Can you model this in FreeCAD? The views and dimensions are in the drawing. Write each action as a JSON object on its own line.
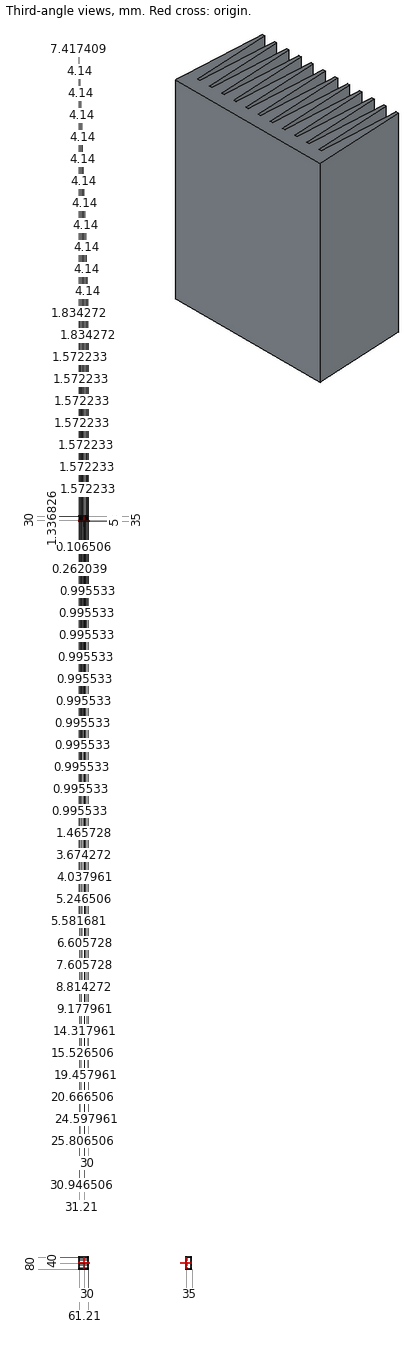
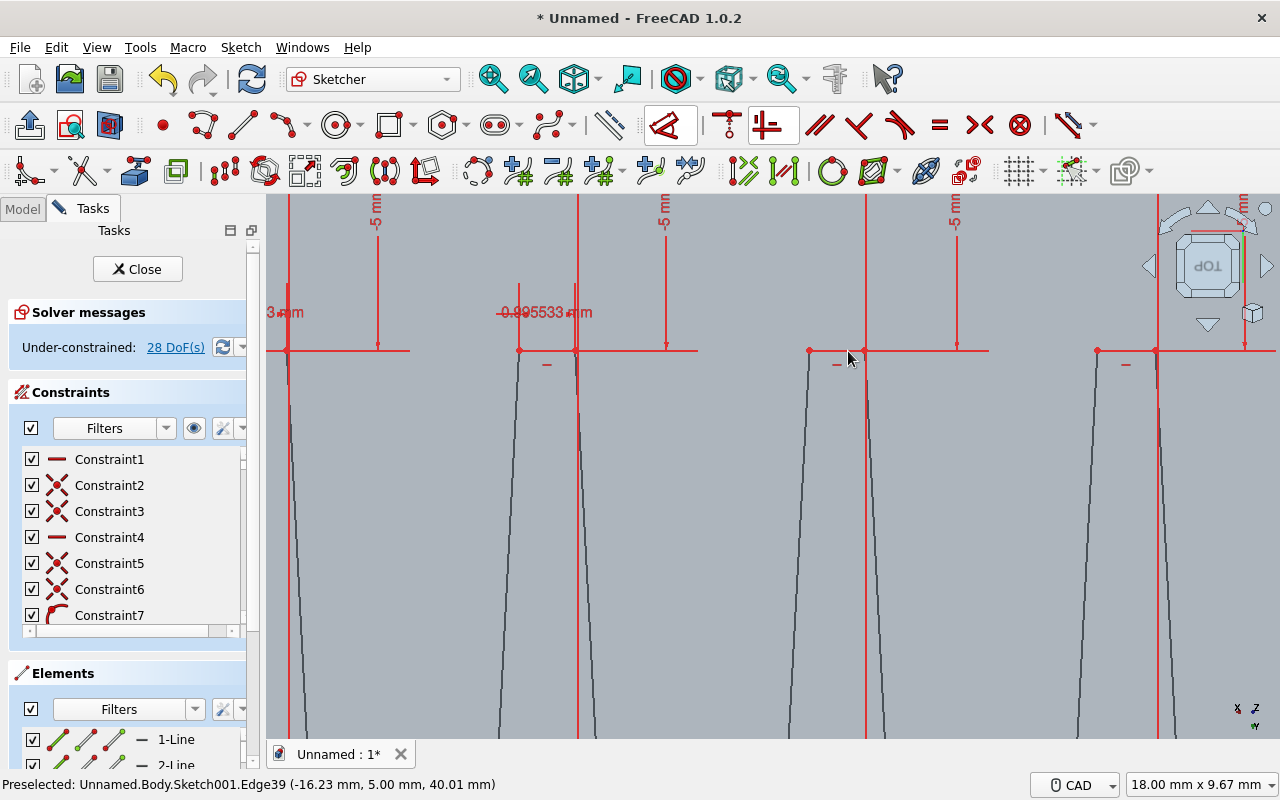
{"action": "key", "text": "l"}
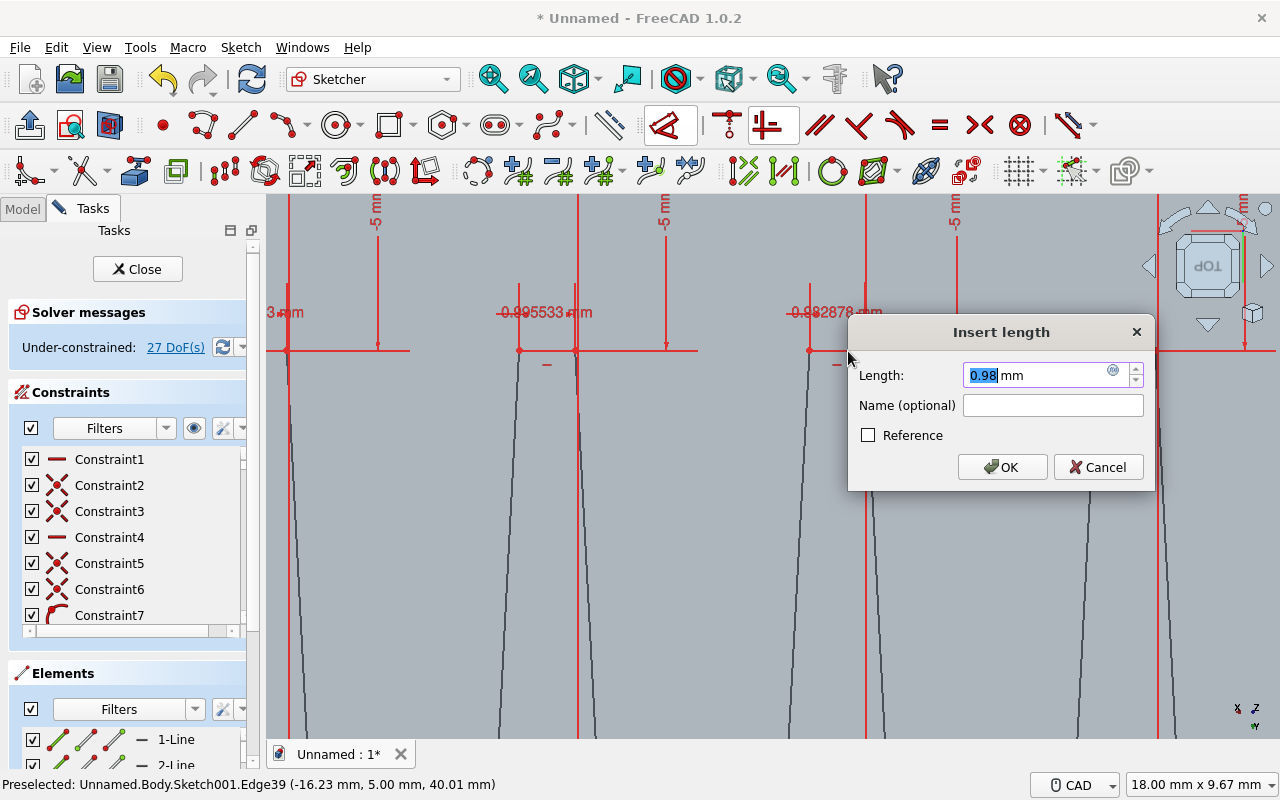
{"action": "type", "text": "0.995533"}
{"action": "key", "text": "Return"}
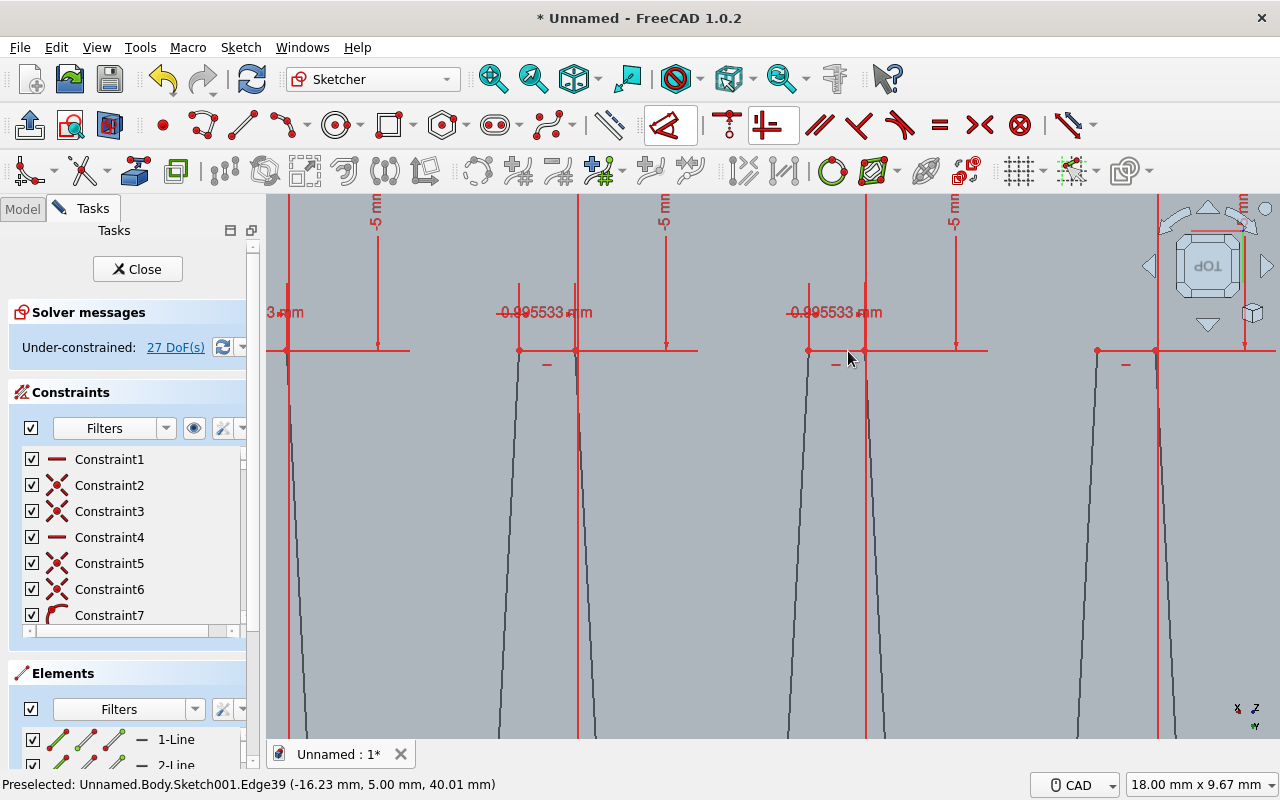
{"action": "left_click", "coordinate": [1115, 351]}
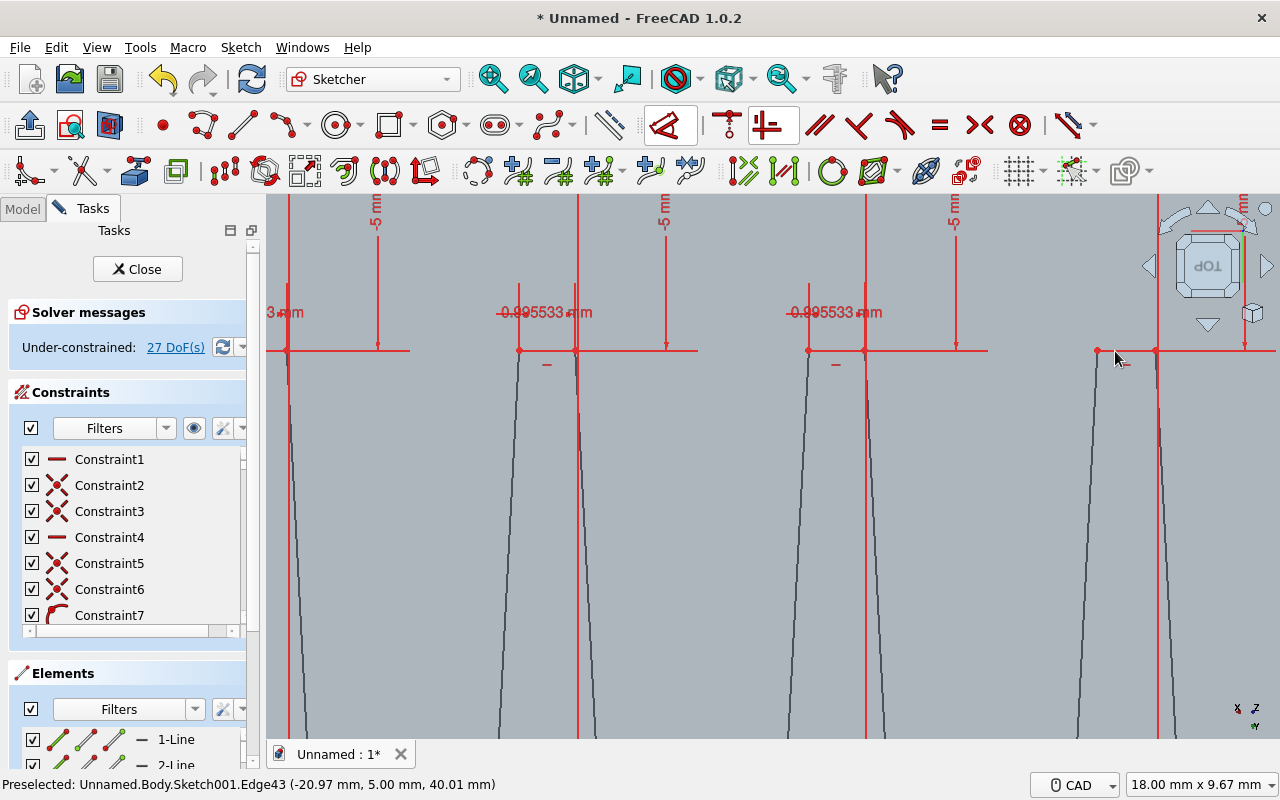
{"action": "key", "text": "l"}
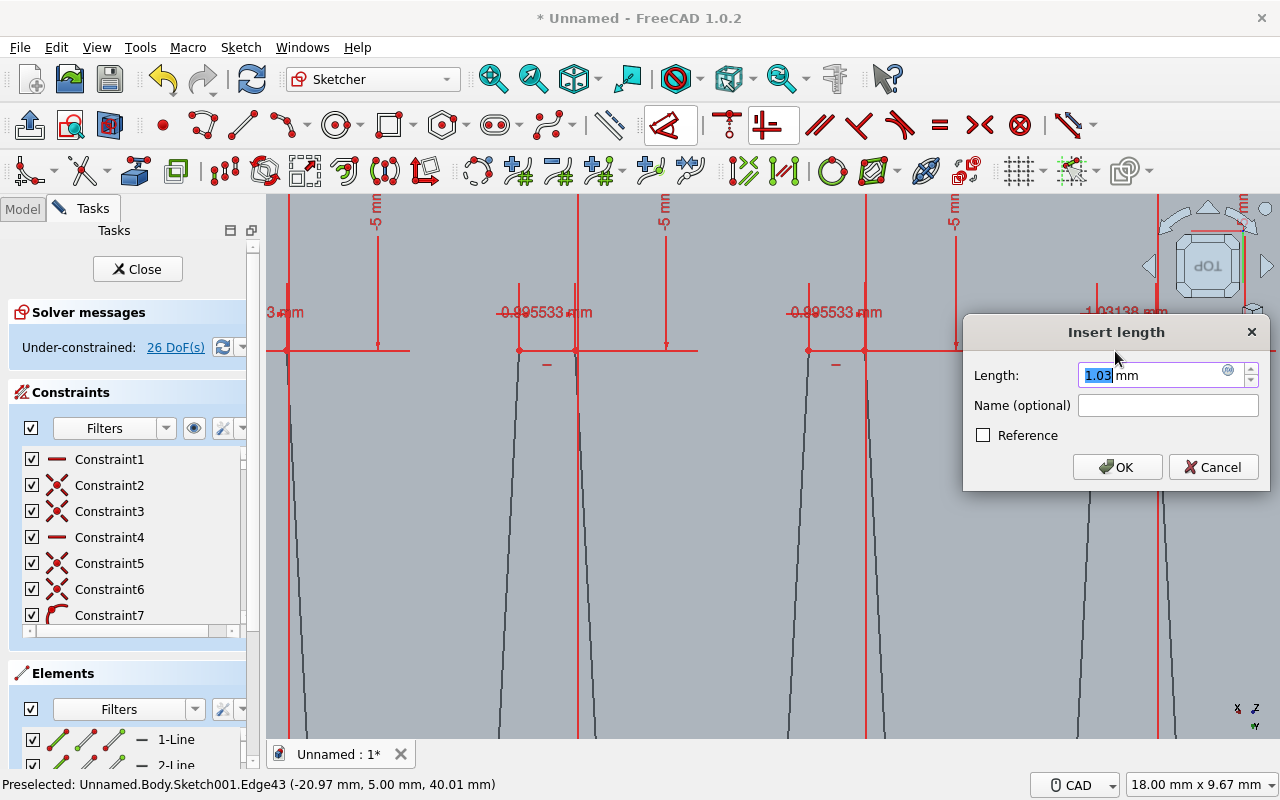
{"action": "type", "text": "0.995533"}
{"action": "key", "text": "Return"}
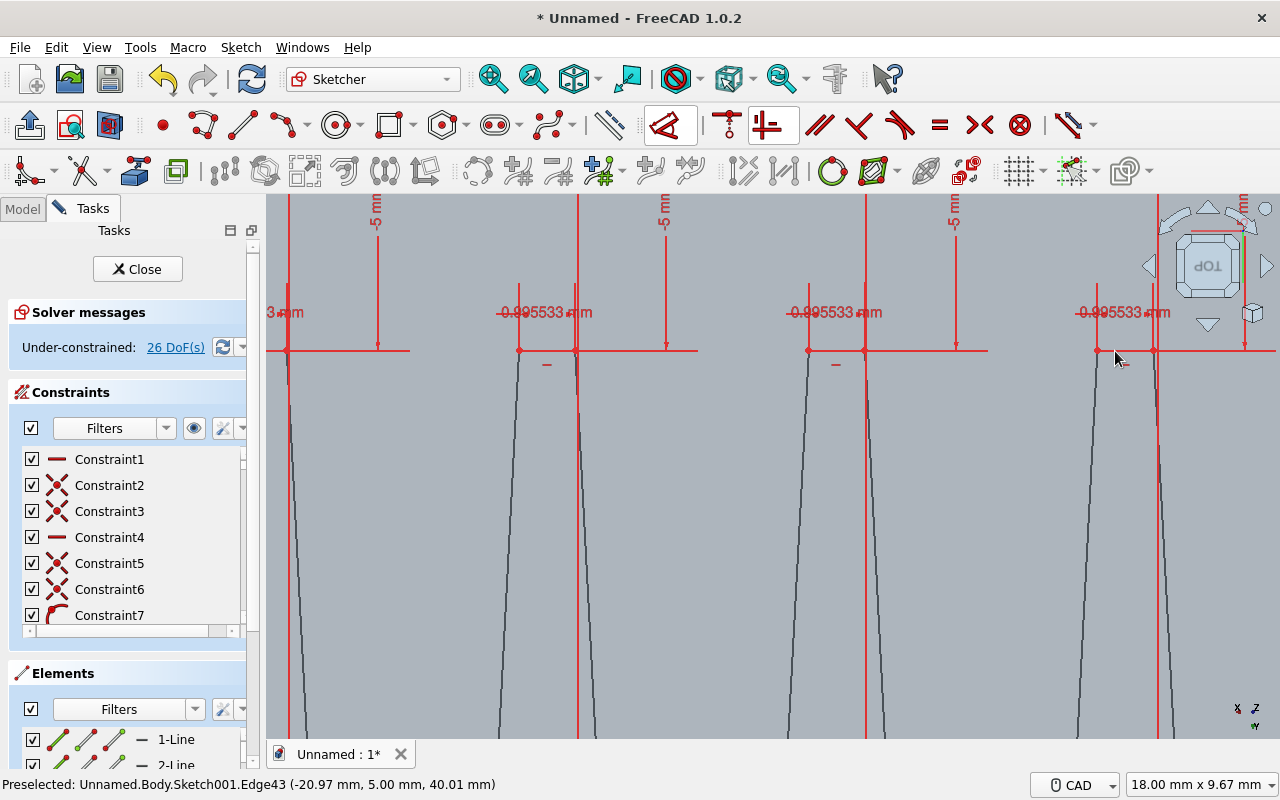
{"action": "scroll", "coordinate": [850, 350], "scroll_direction": "down", "scroll_amount": 9}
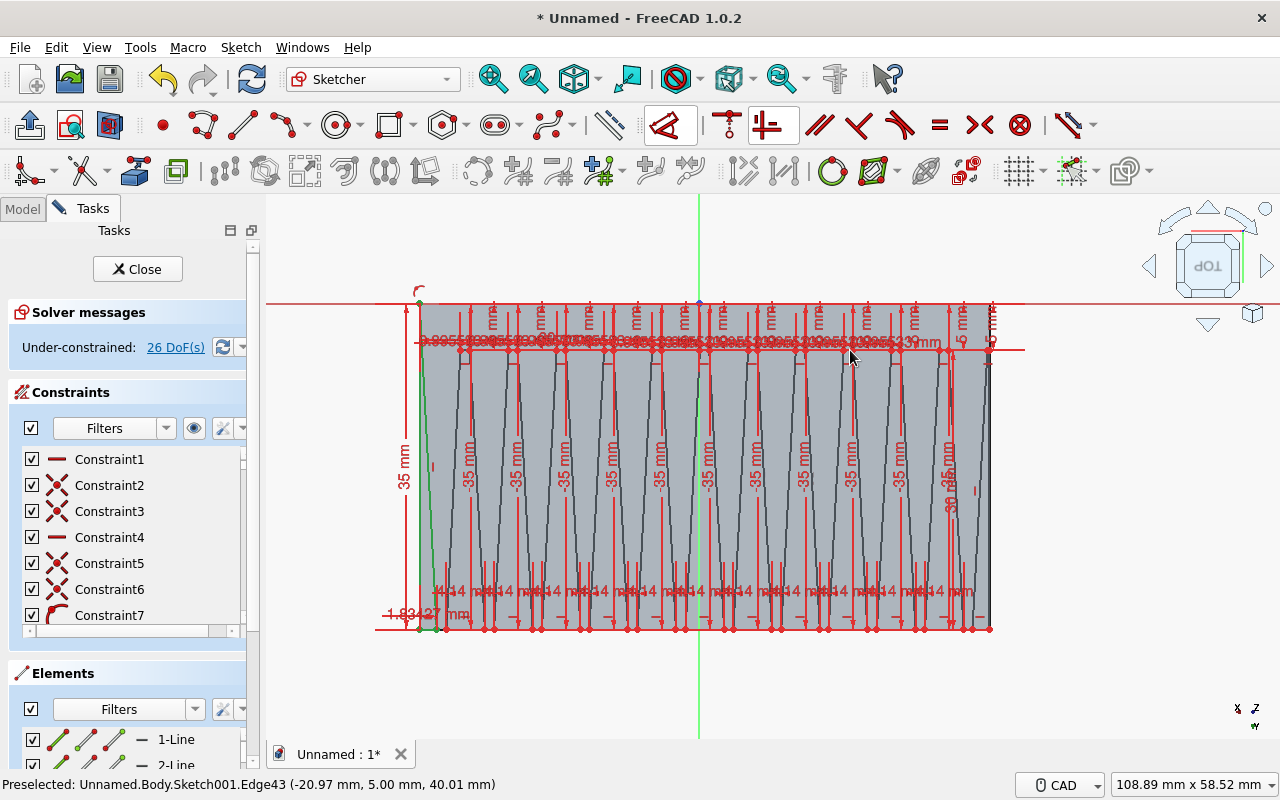
{"action": "scroll", "coordinate": [946, 350], "scroll_direction": "up", "scroll_amount": 9}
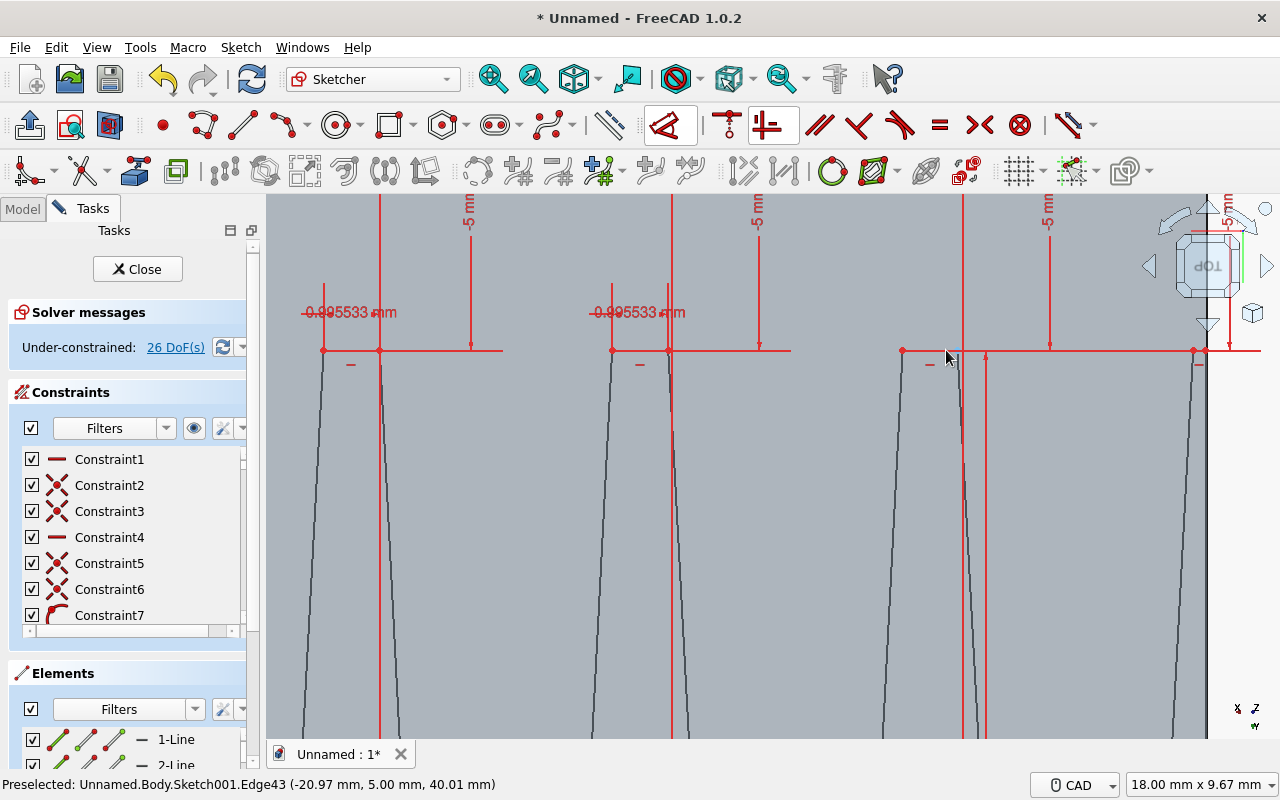
{"action": "left_click", "coordinate": [941, 351]}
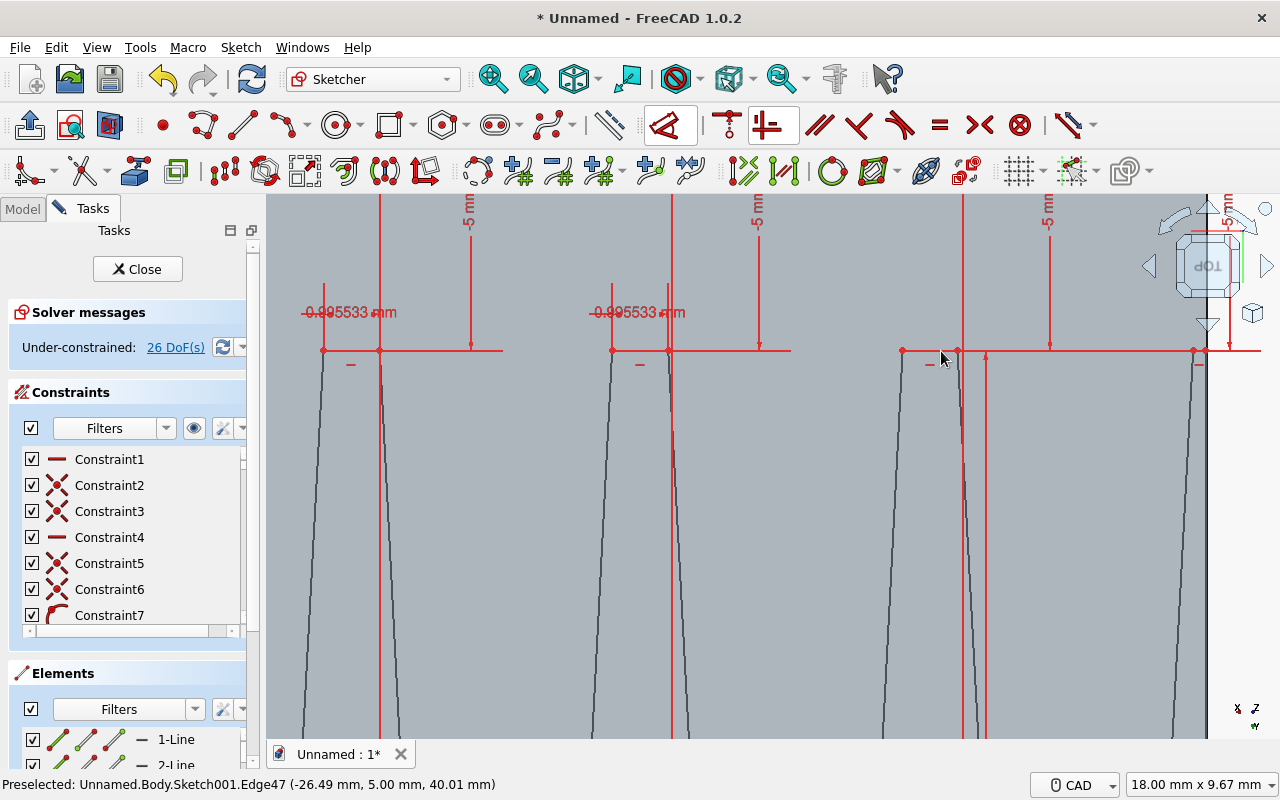
{"action": "left_click", "coordinate": [692, 126]}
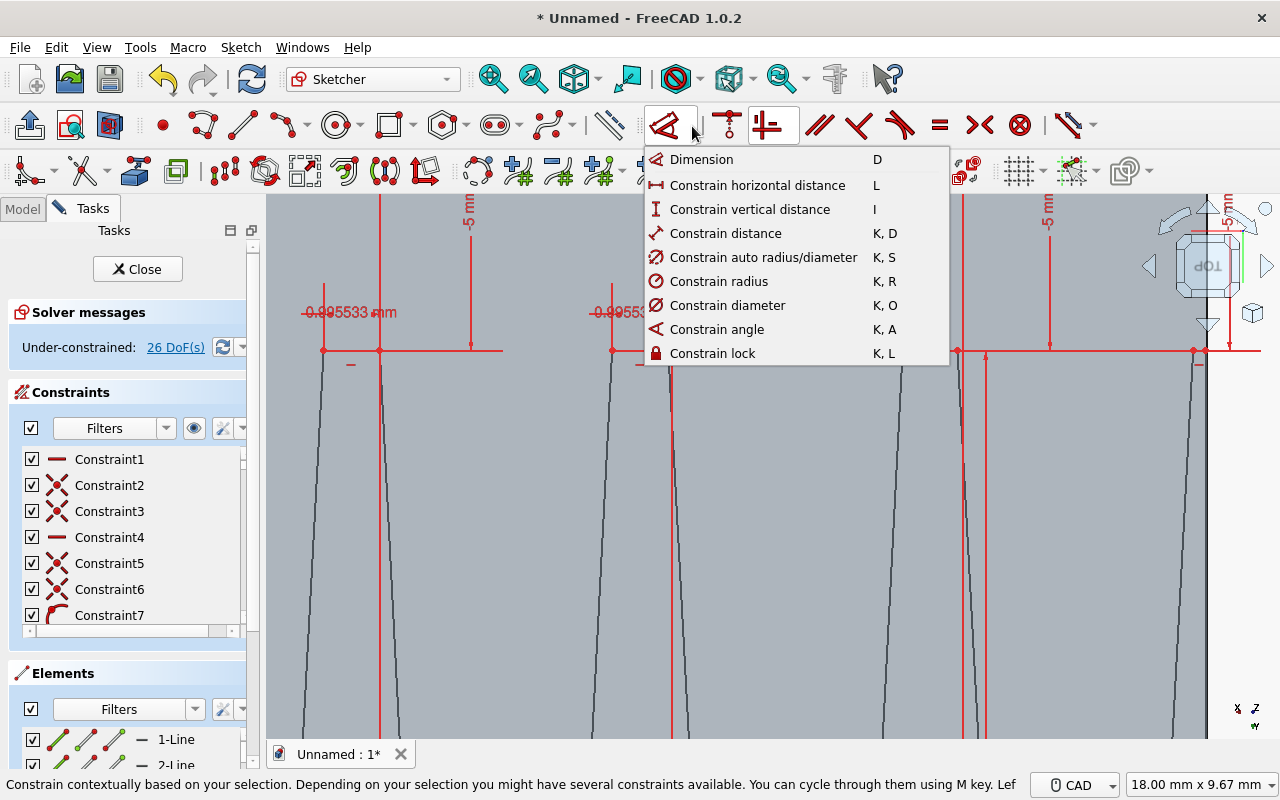
{"action": "left_click", "coordinate": [797, 185]}